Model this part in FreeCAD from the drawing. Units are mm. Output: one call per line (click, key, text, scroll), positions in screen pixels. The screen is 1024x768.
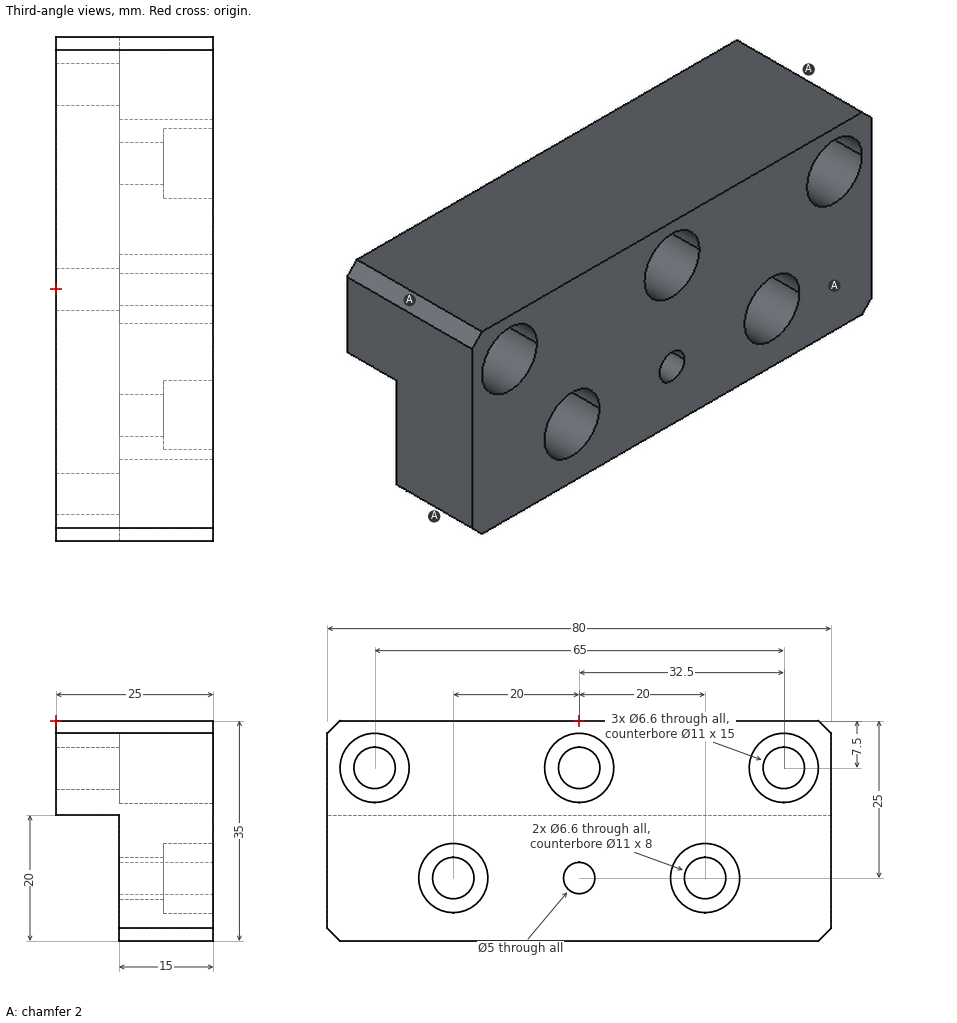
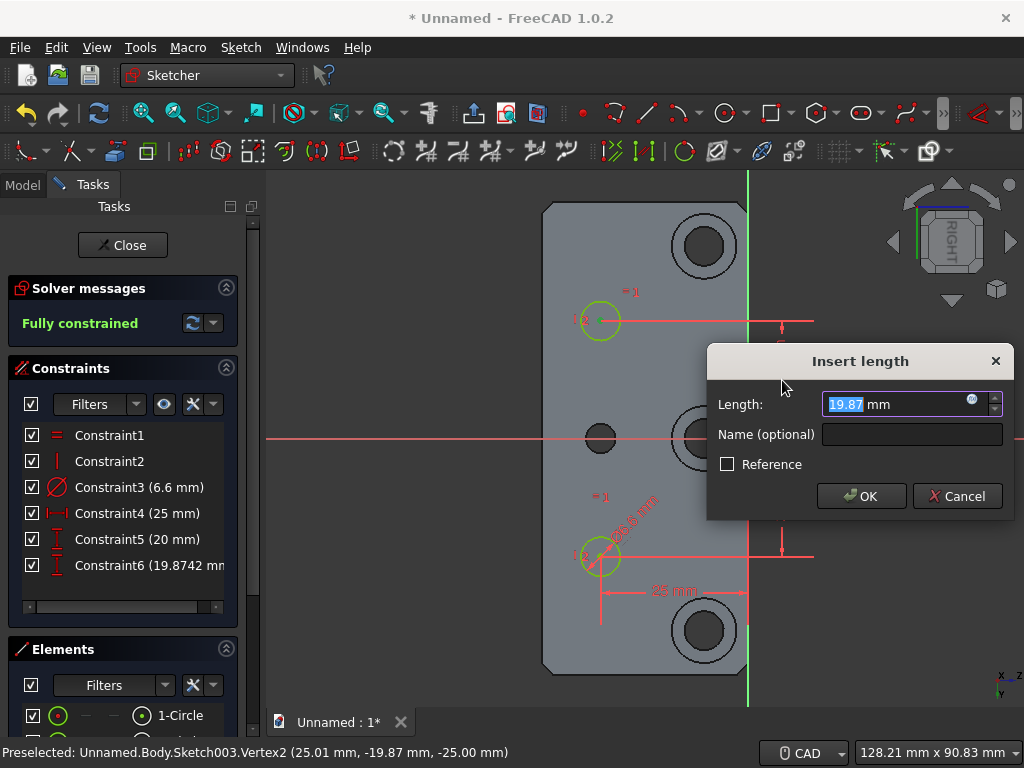
text(20)
key(Return)
key(Escape)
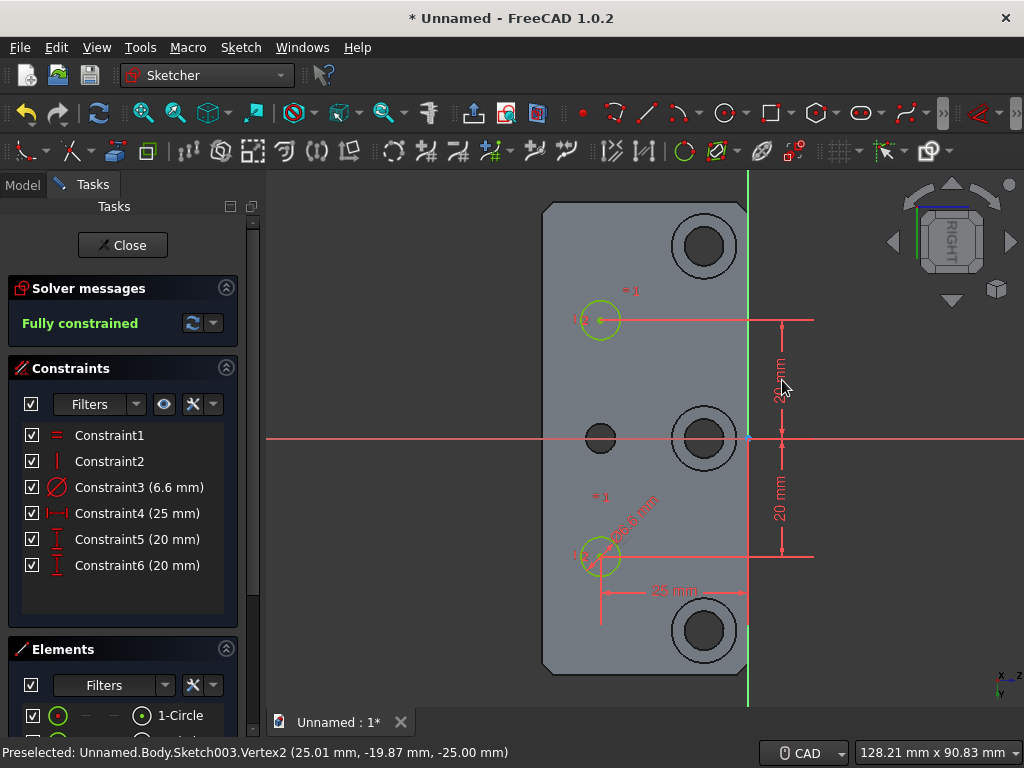
click(123, 245)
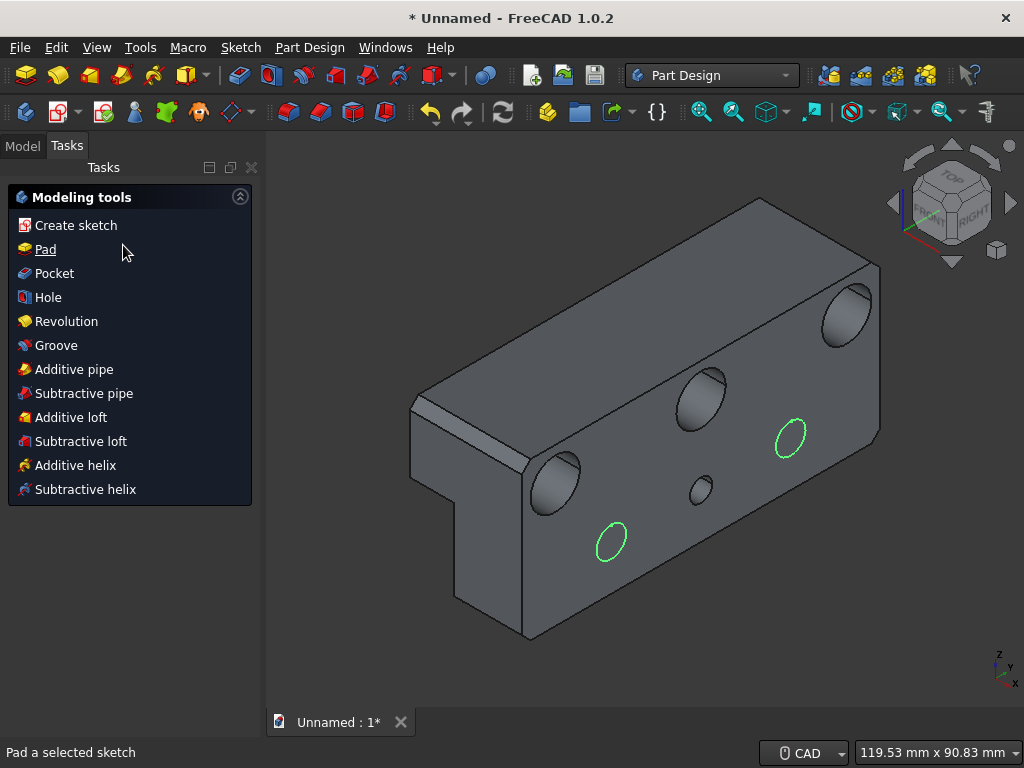
click(272, 76)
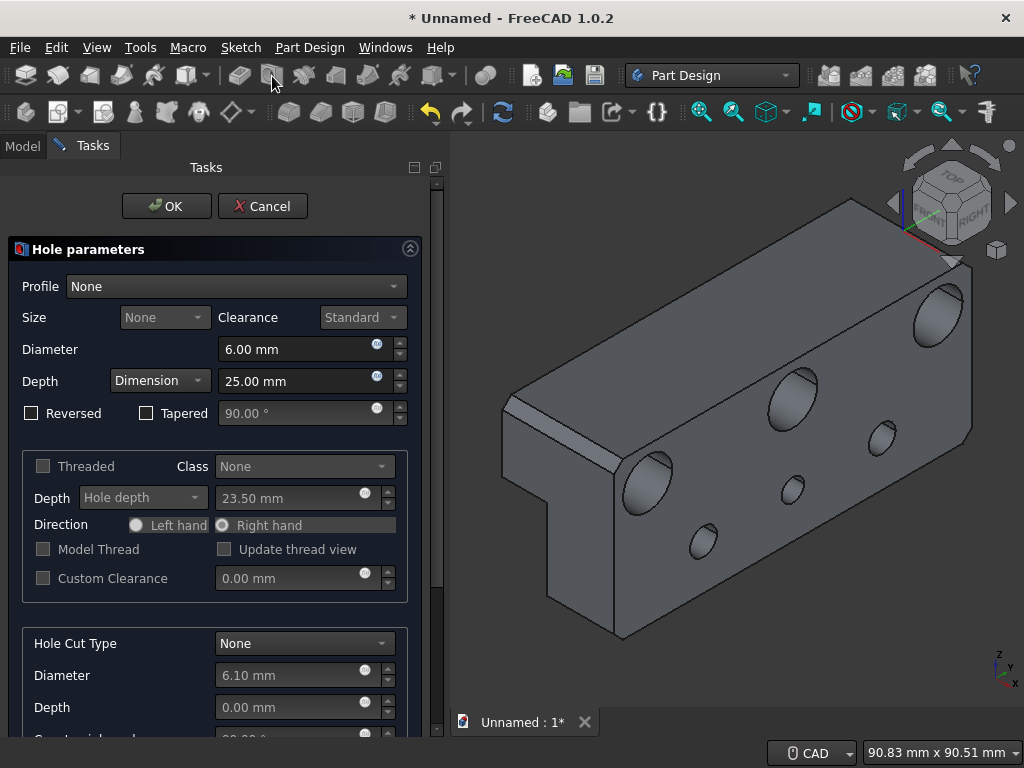
triple_click(305, 349)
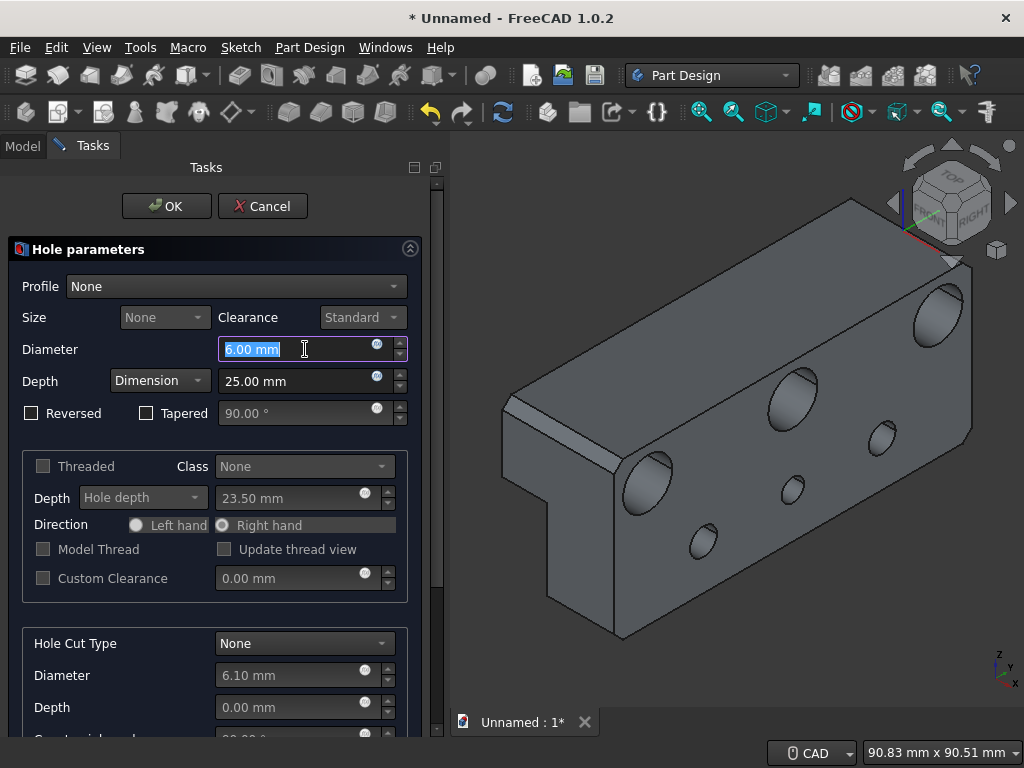
text(6.6)
key(Tab)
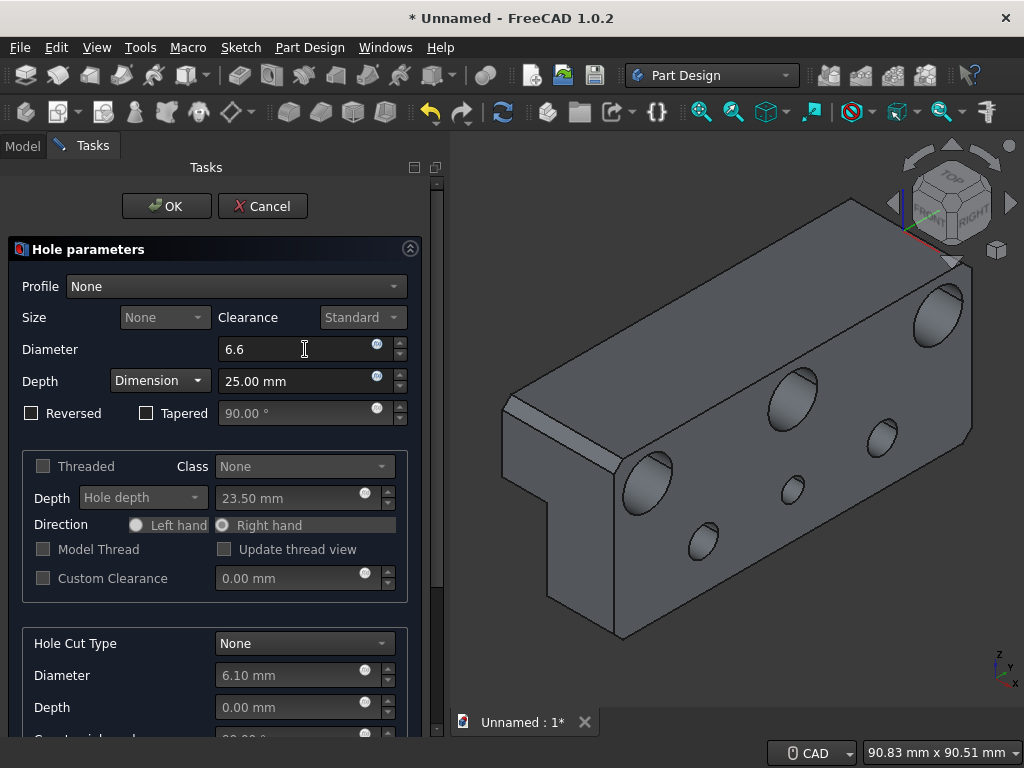
click(161, 380)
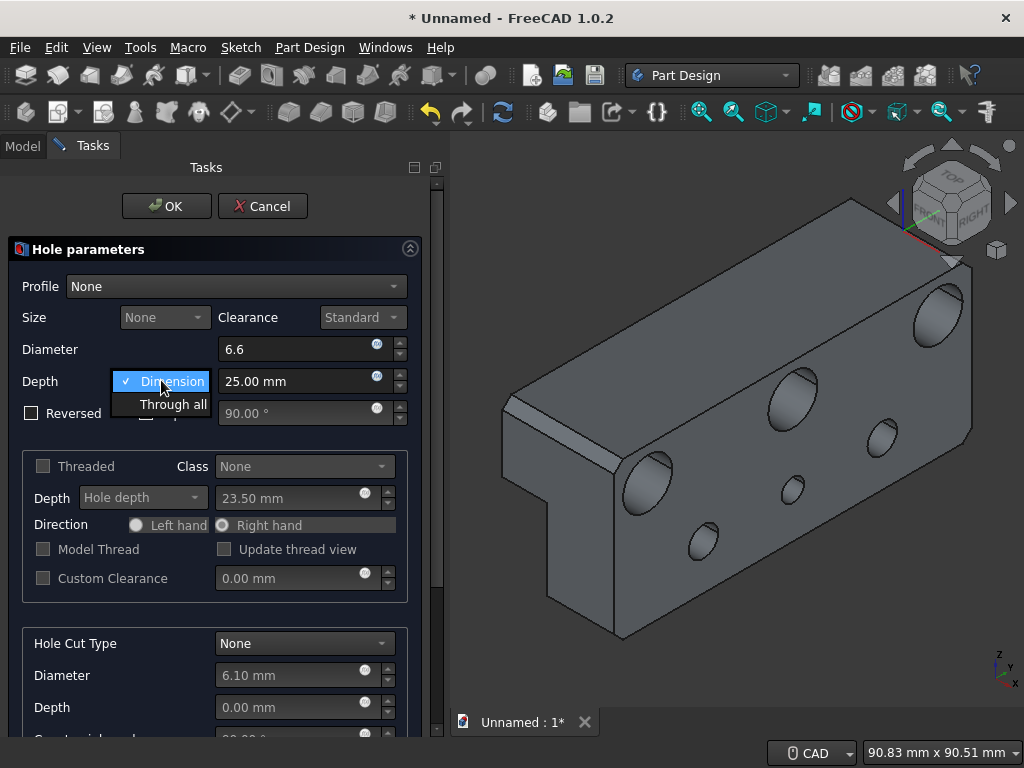
click(160, 404)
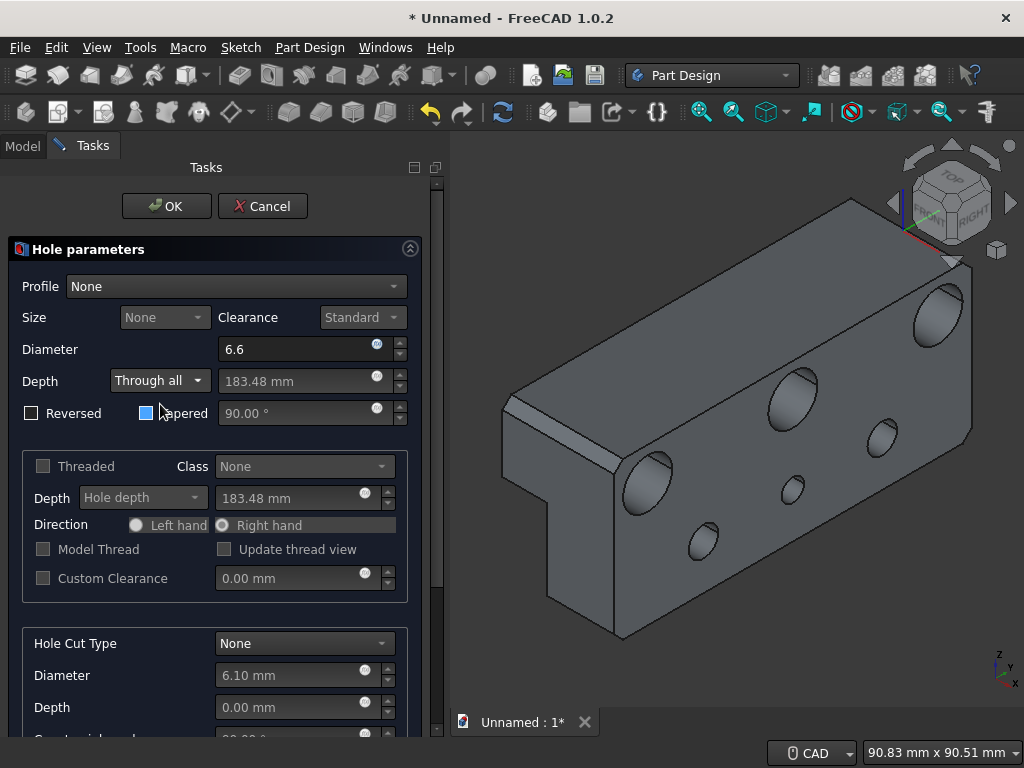
click(306, 644)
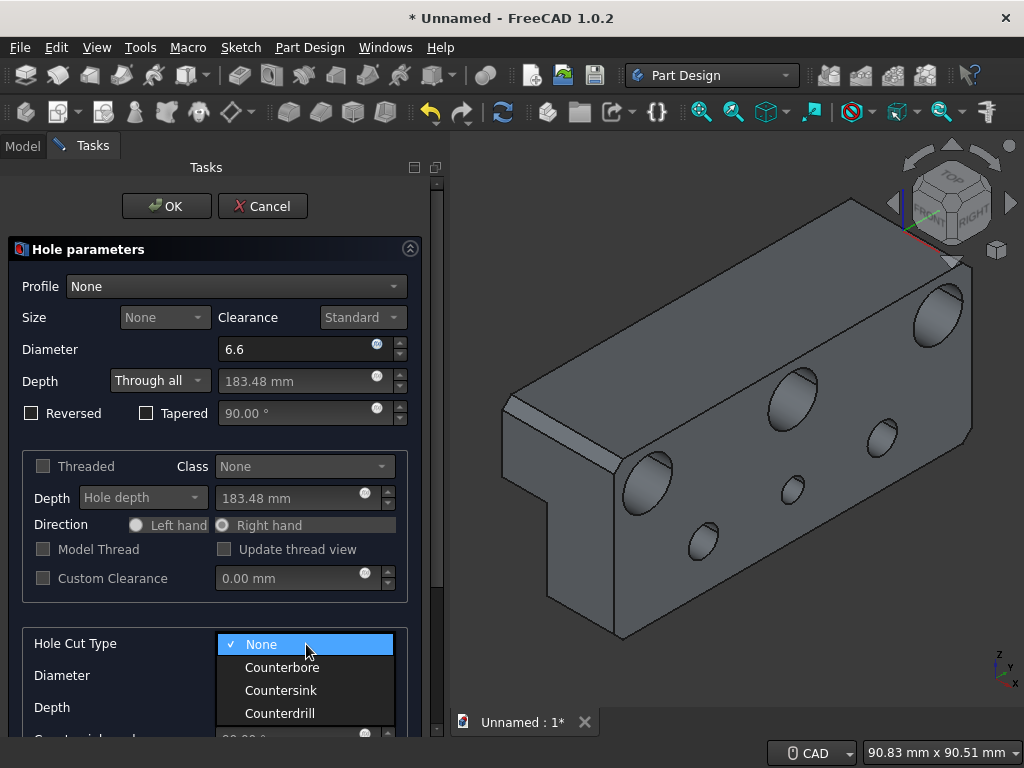
click(304, 668)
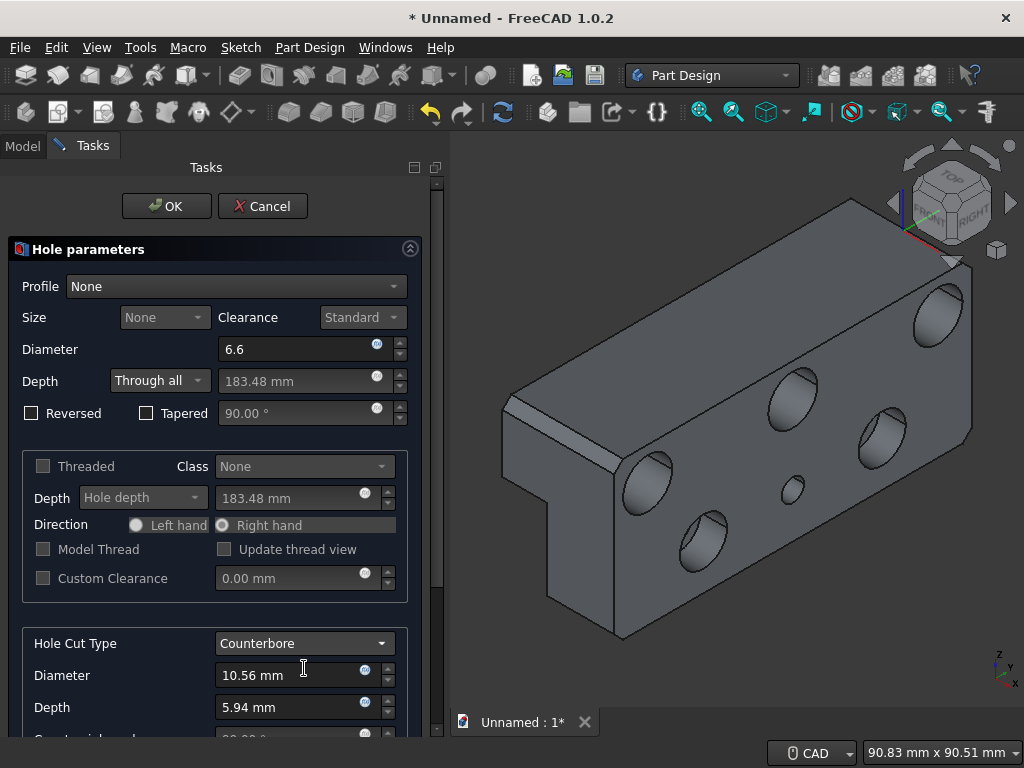
triple_click(298, 675)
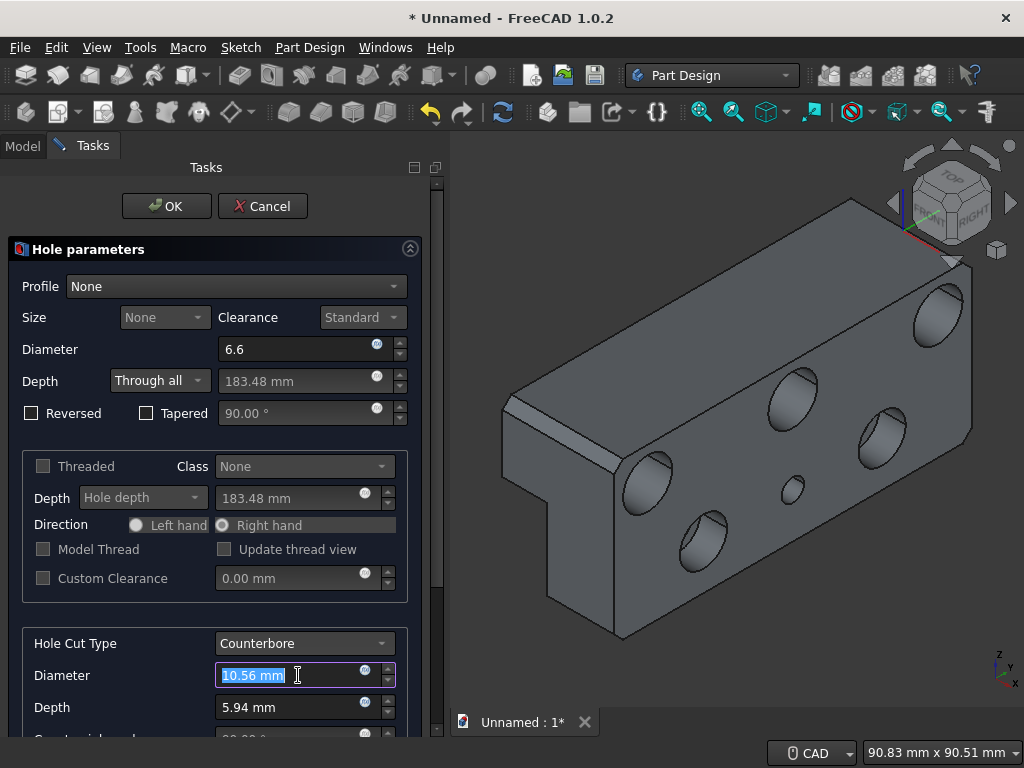
text(11)
key(Tab)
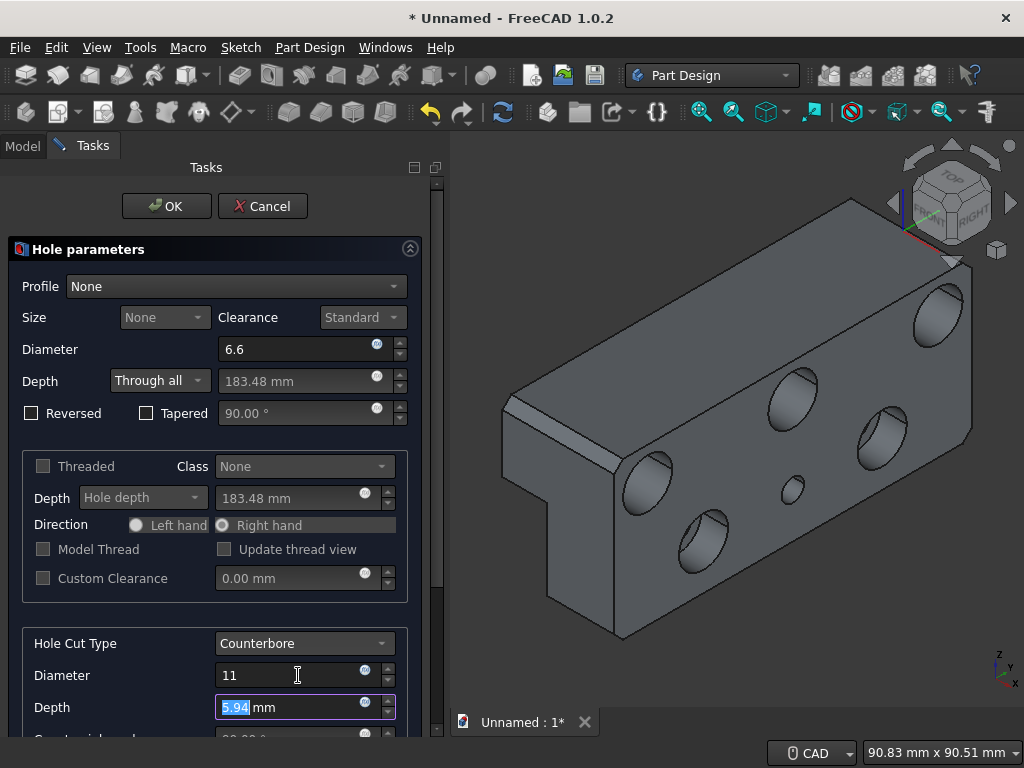
text(8)
key(Tab)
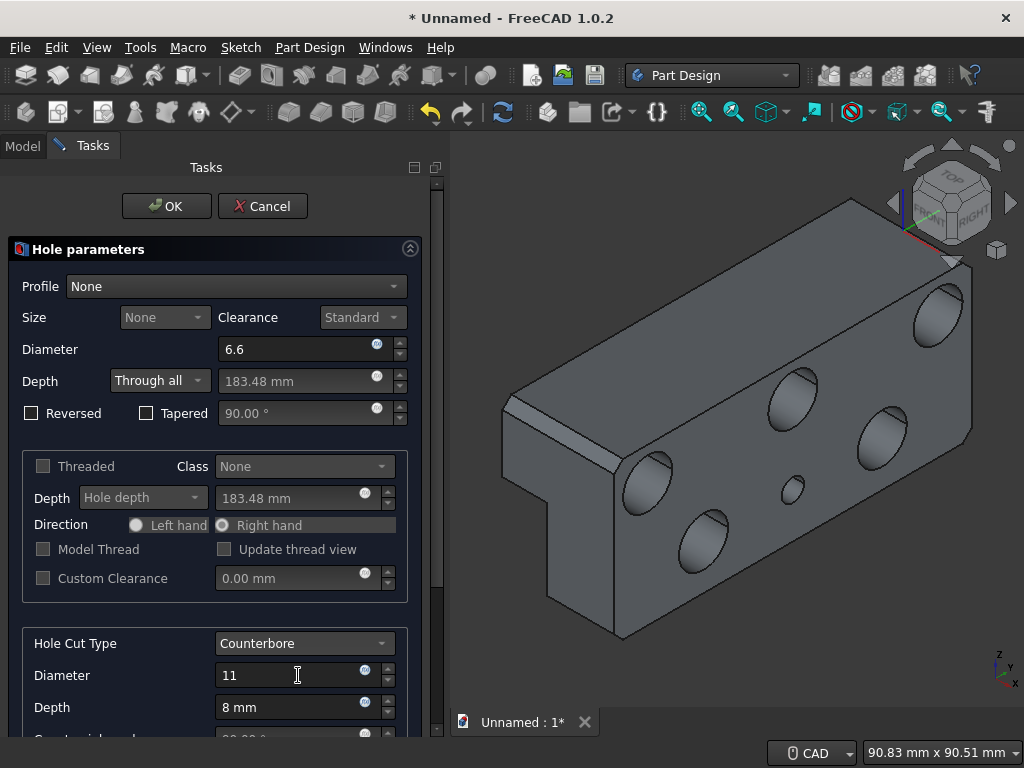
click(167, 206)